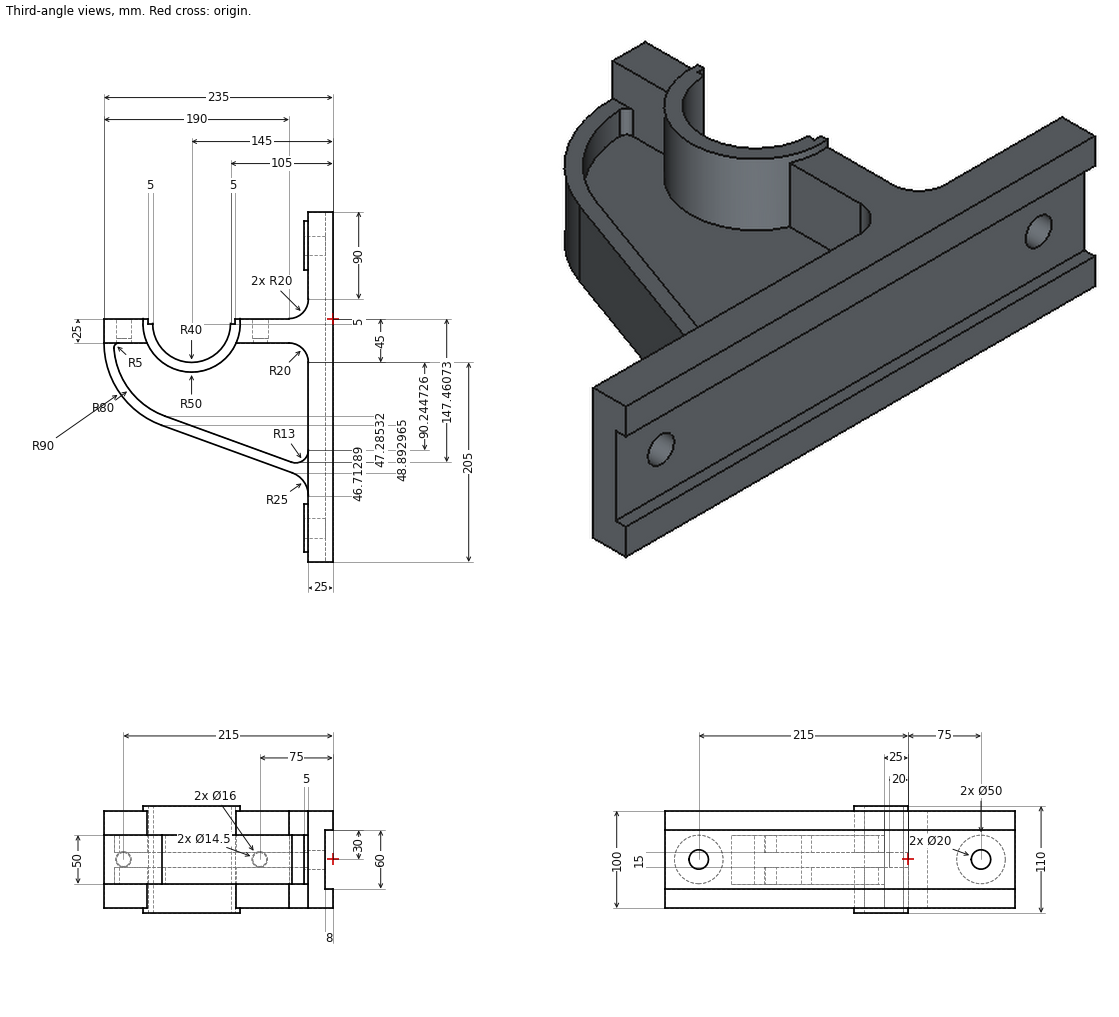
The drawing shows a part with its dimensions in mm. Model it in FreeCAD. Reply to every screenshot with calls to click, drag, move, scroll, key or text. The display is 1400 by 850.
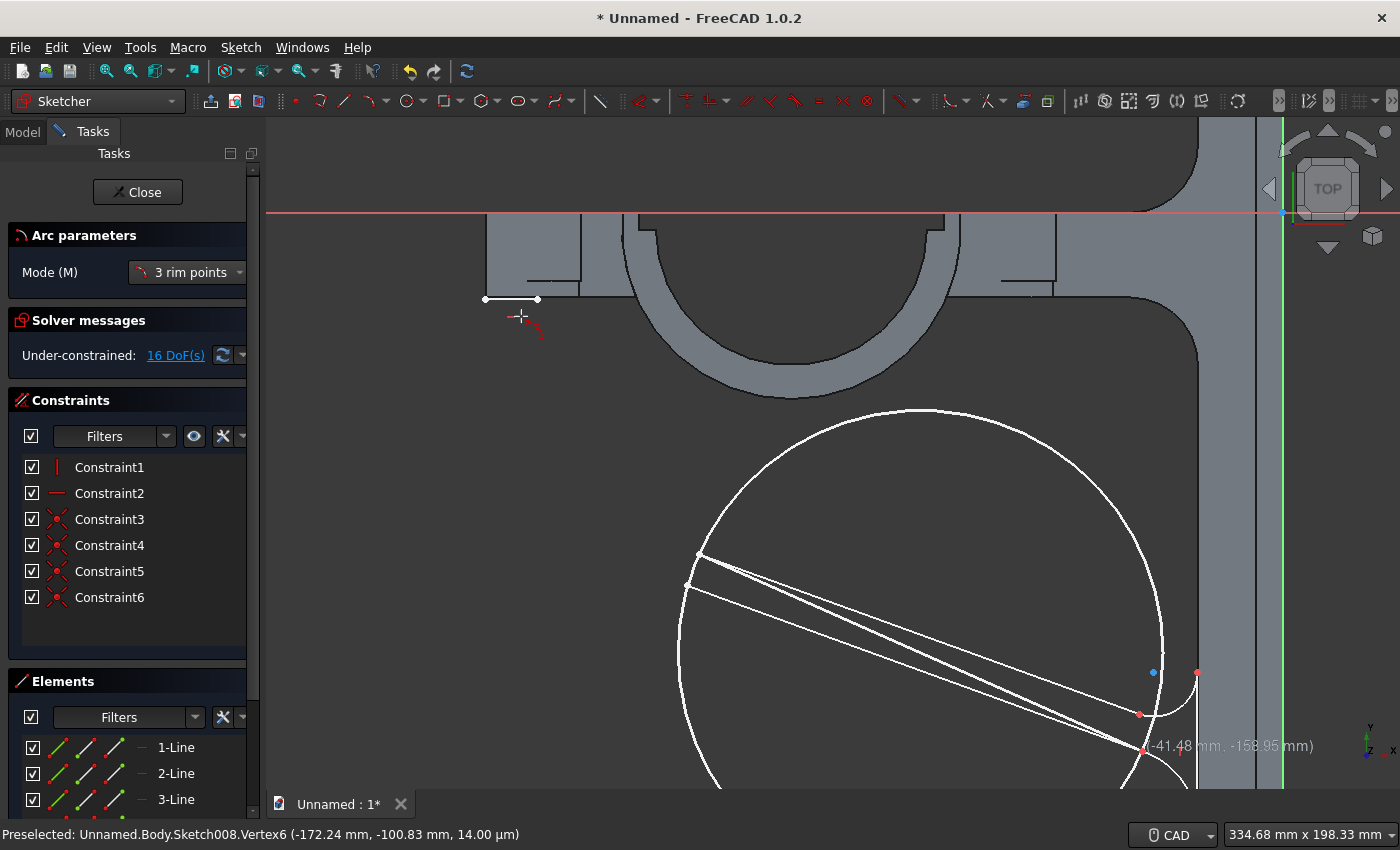
click(521, 316)
click(575, 460)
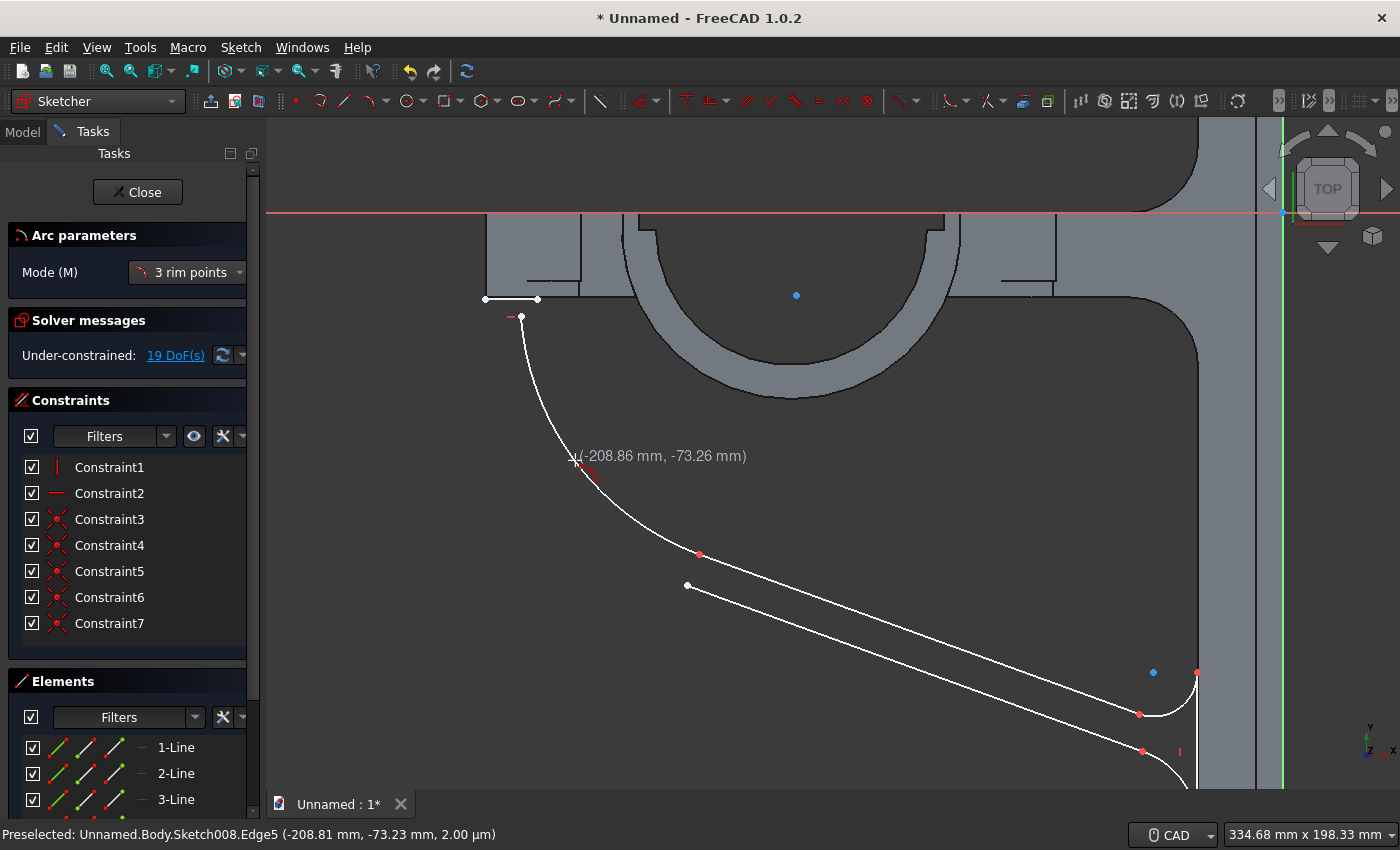
click(521, 317)
click(538, 299)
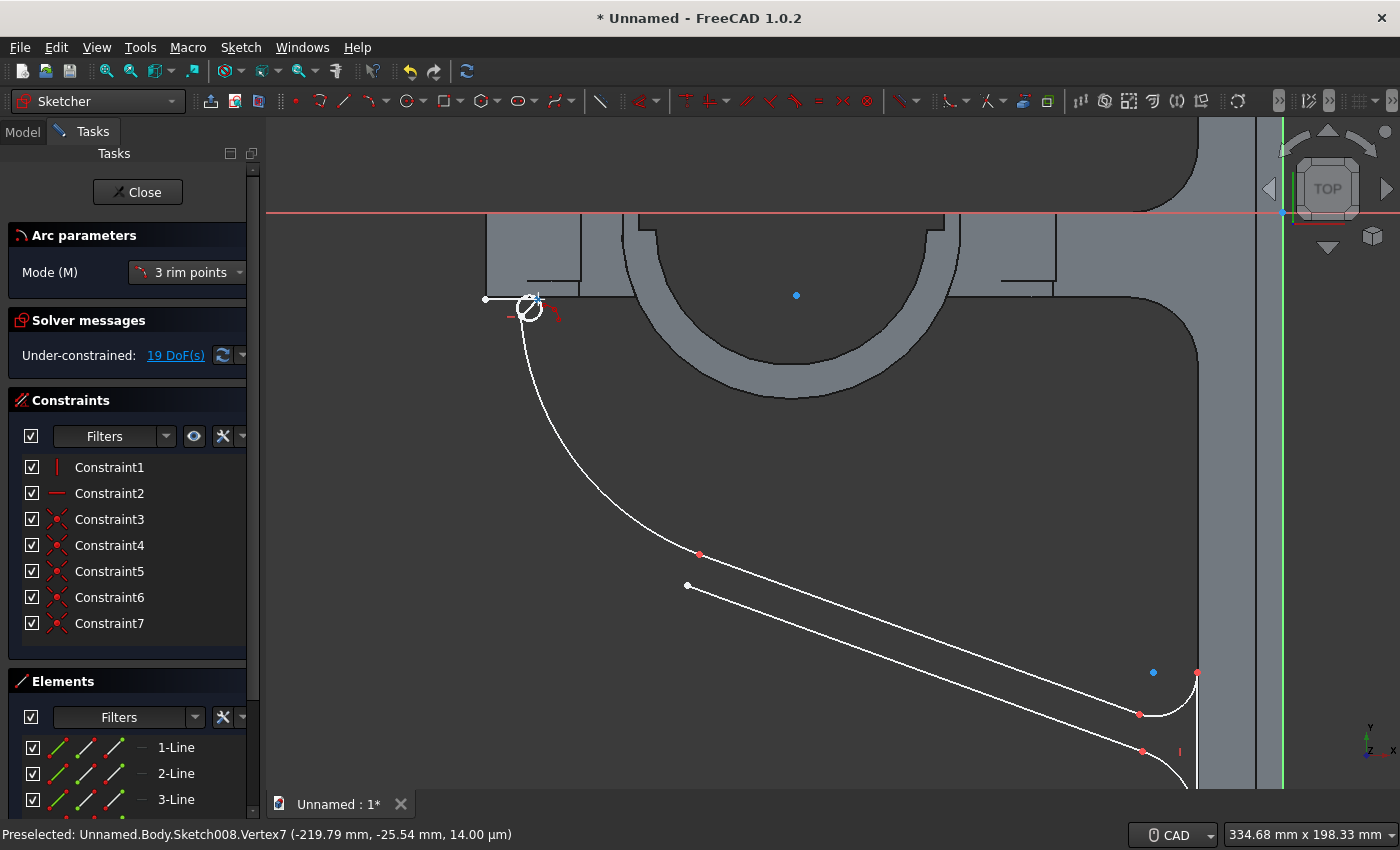
scroll(525, 303, up, 6)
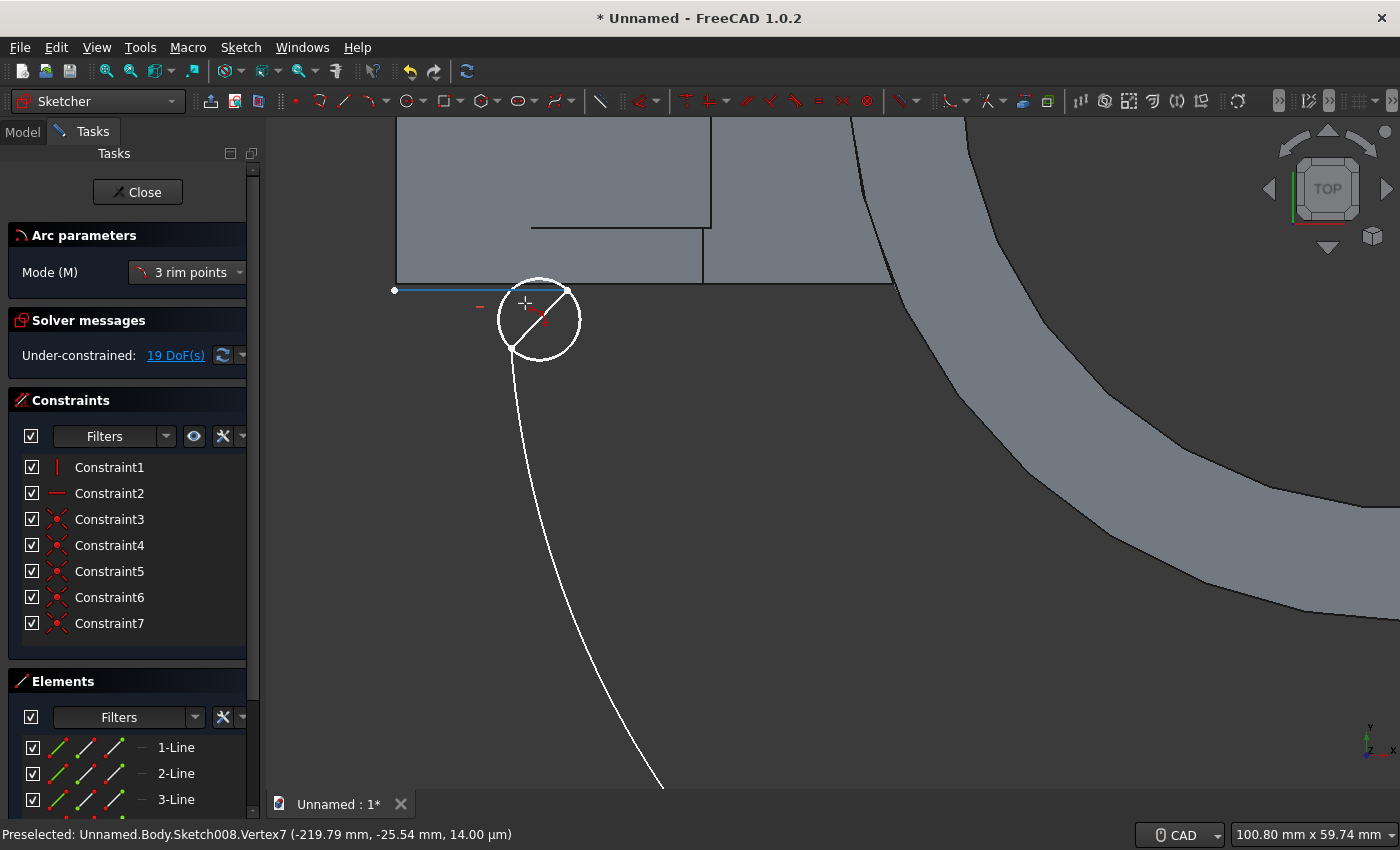
click(526, 302)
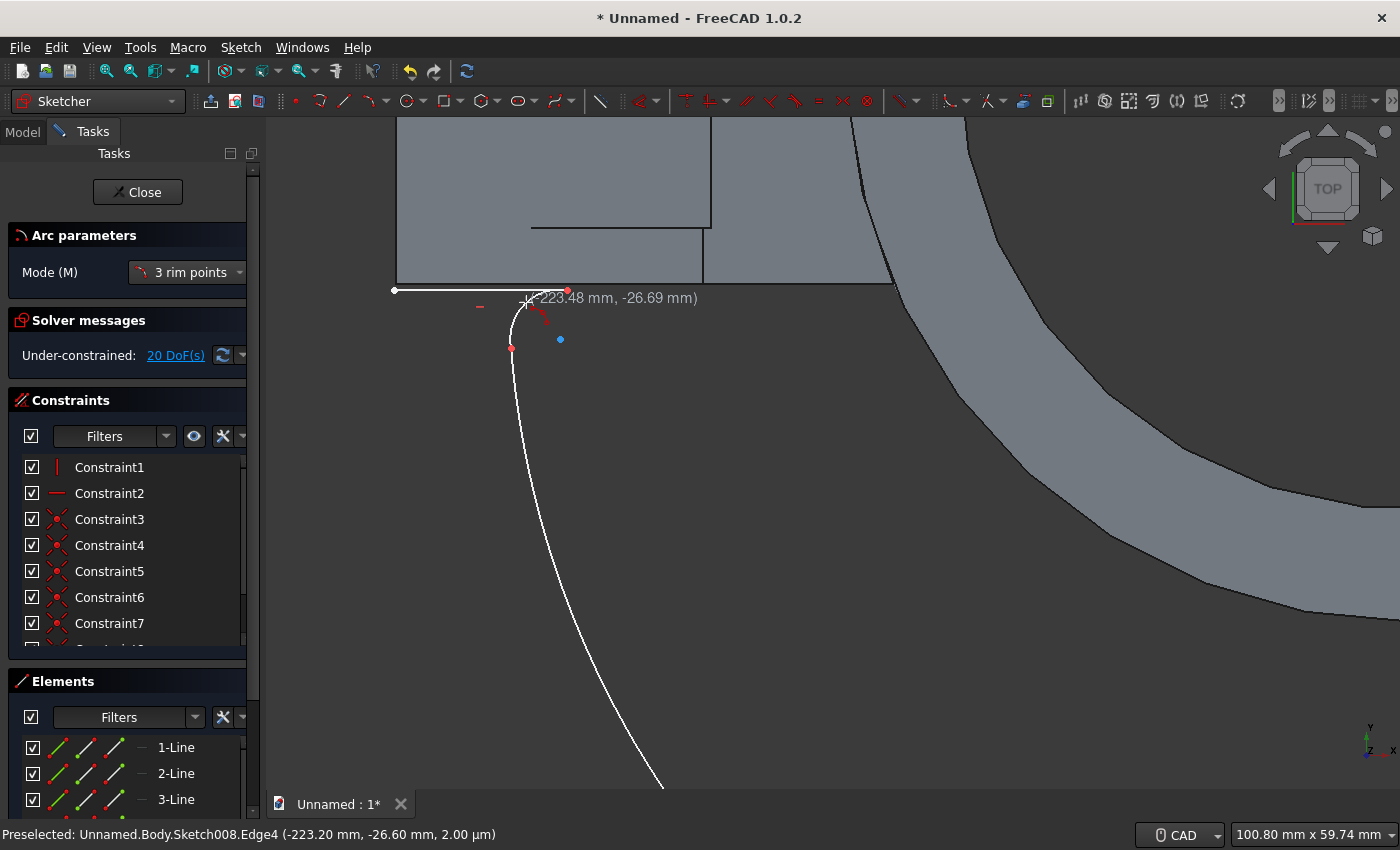
scroll(523, 308, down, 8)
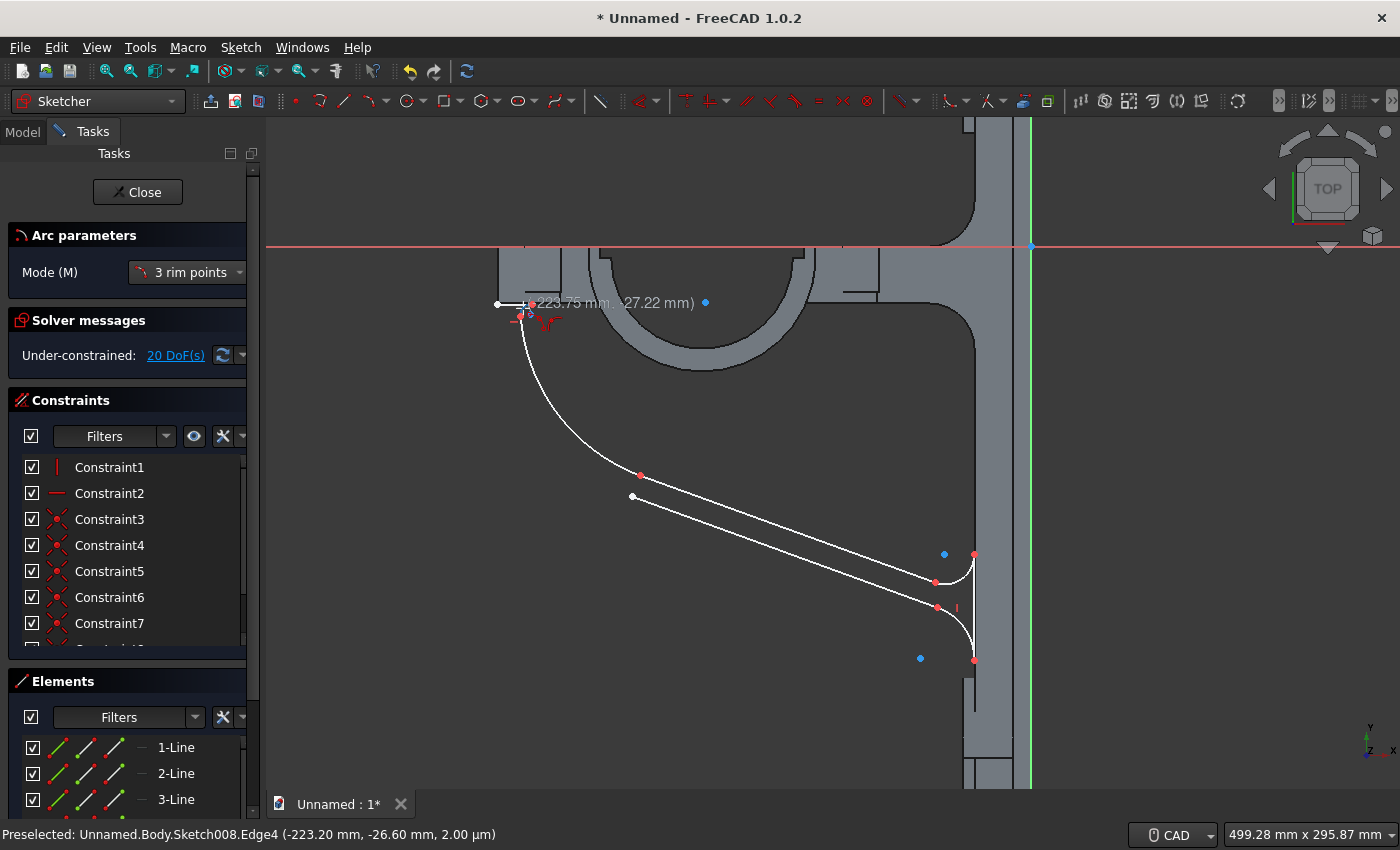
click(497, 305)
click(632, 497)
click(535, 421)
key(Escape)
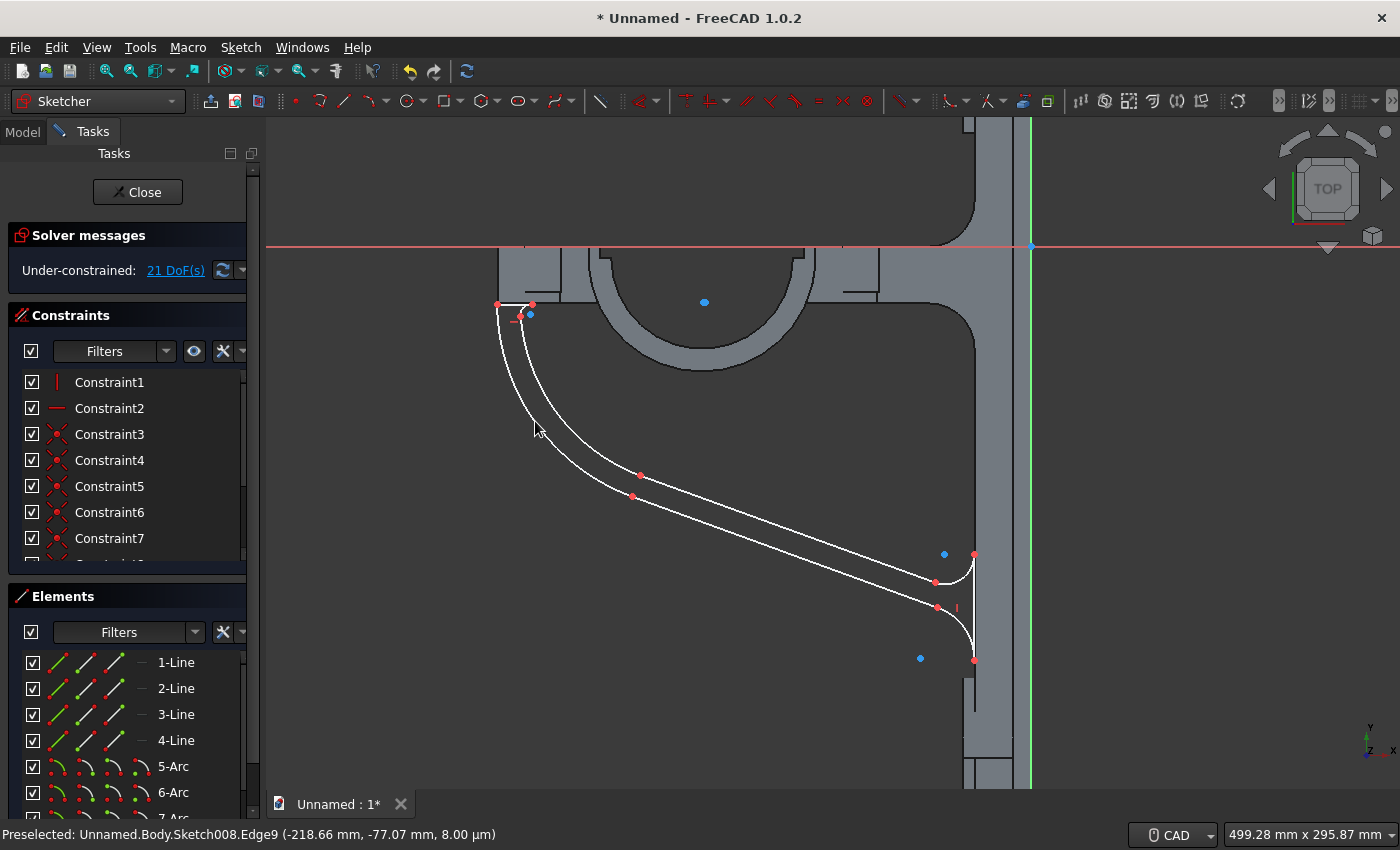
click(724, 530)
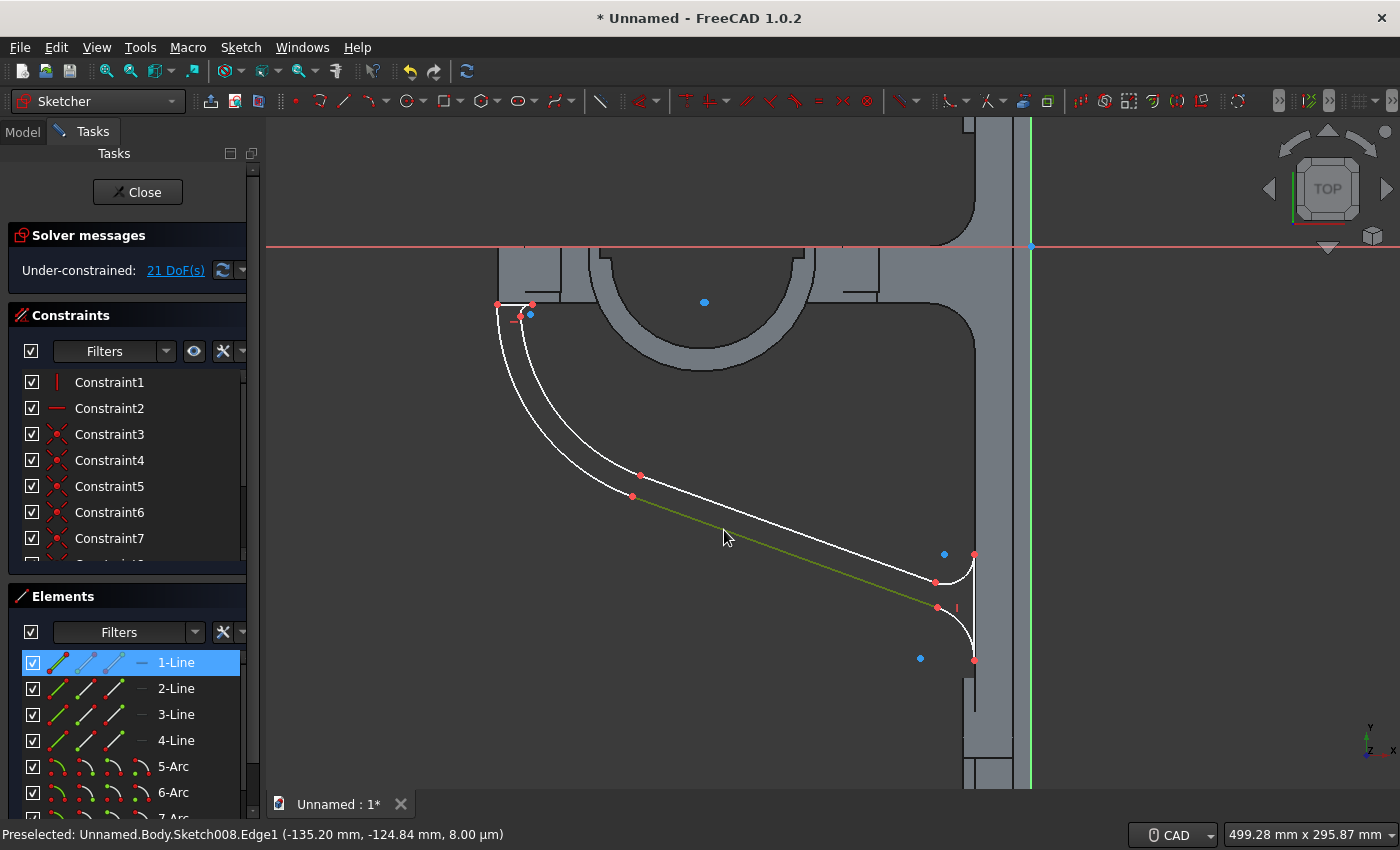
click(955, 618)